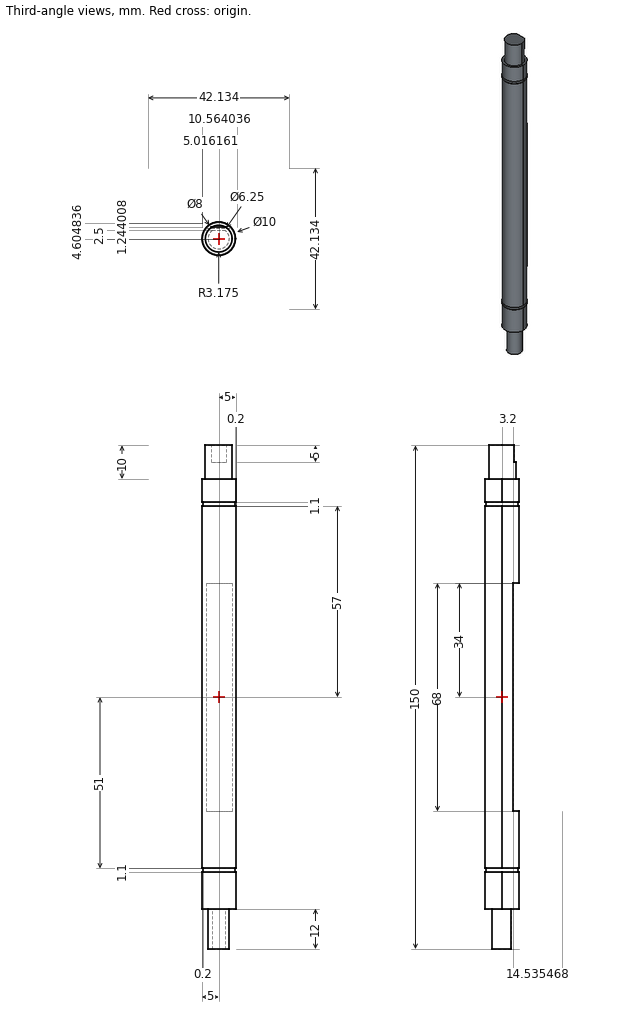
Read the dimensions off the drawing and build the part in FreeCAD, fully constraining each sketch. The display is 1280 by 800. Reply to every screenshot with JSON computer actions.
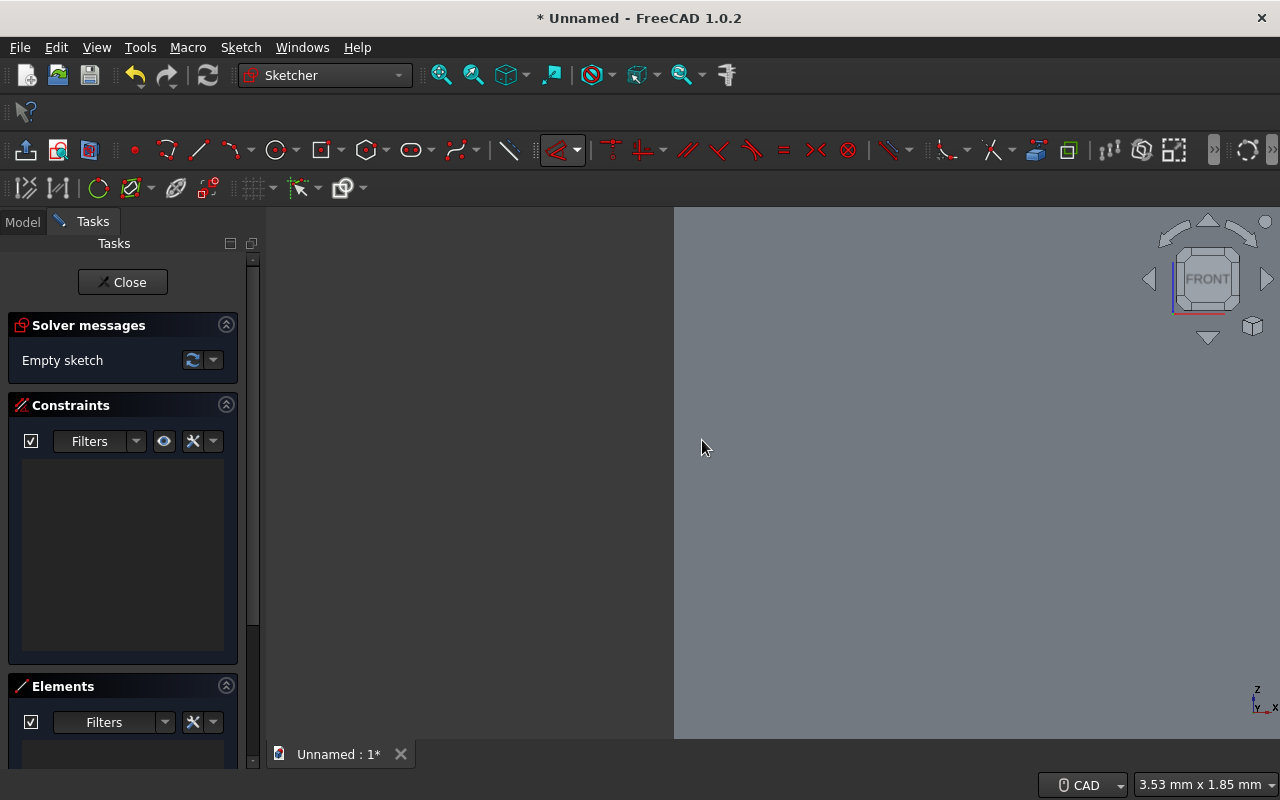
{"action": "left_click", "coordinate": [344, 150]}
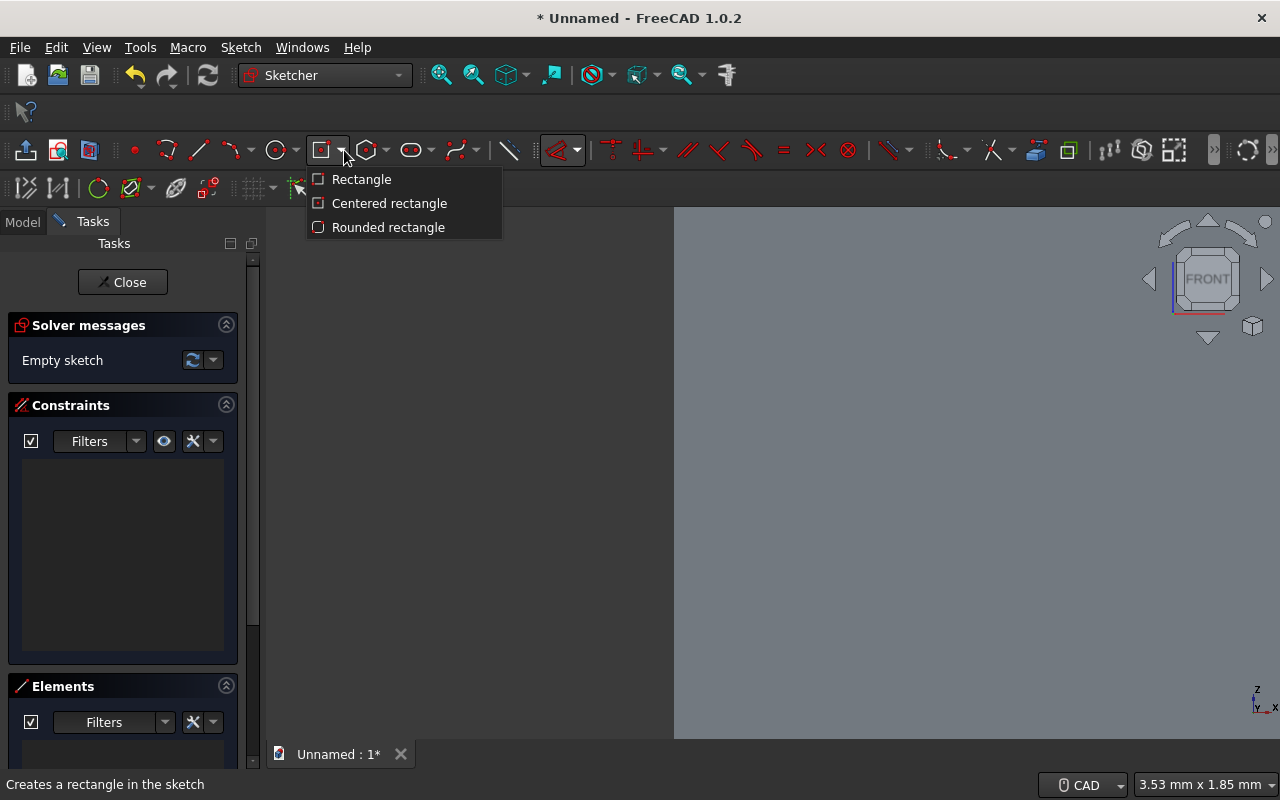
{"action": "left_click", "coordinate": [404, 179]}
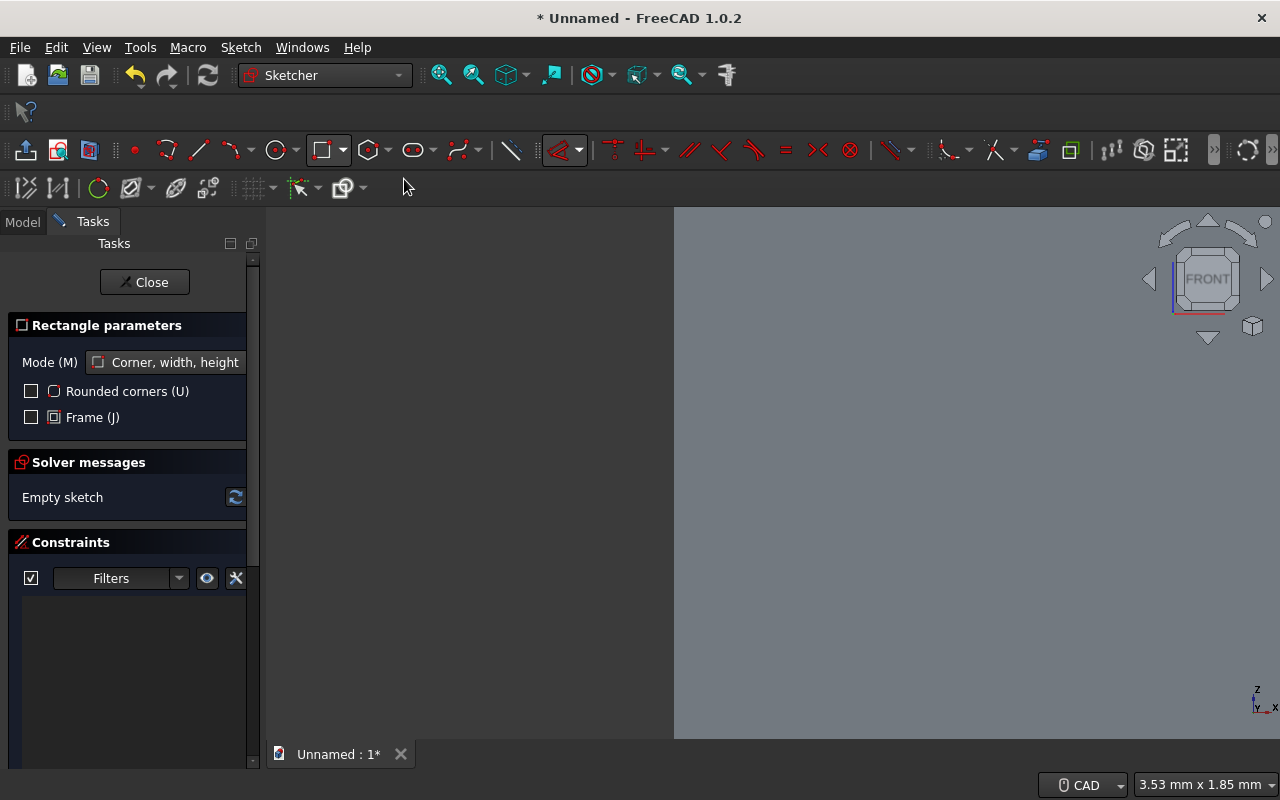
{"action": "left_click", "coordinate": [674, 314]}
{"action": "left_click", "coordinate": [731, 630]}
{"action": "key", "text": "Escape"}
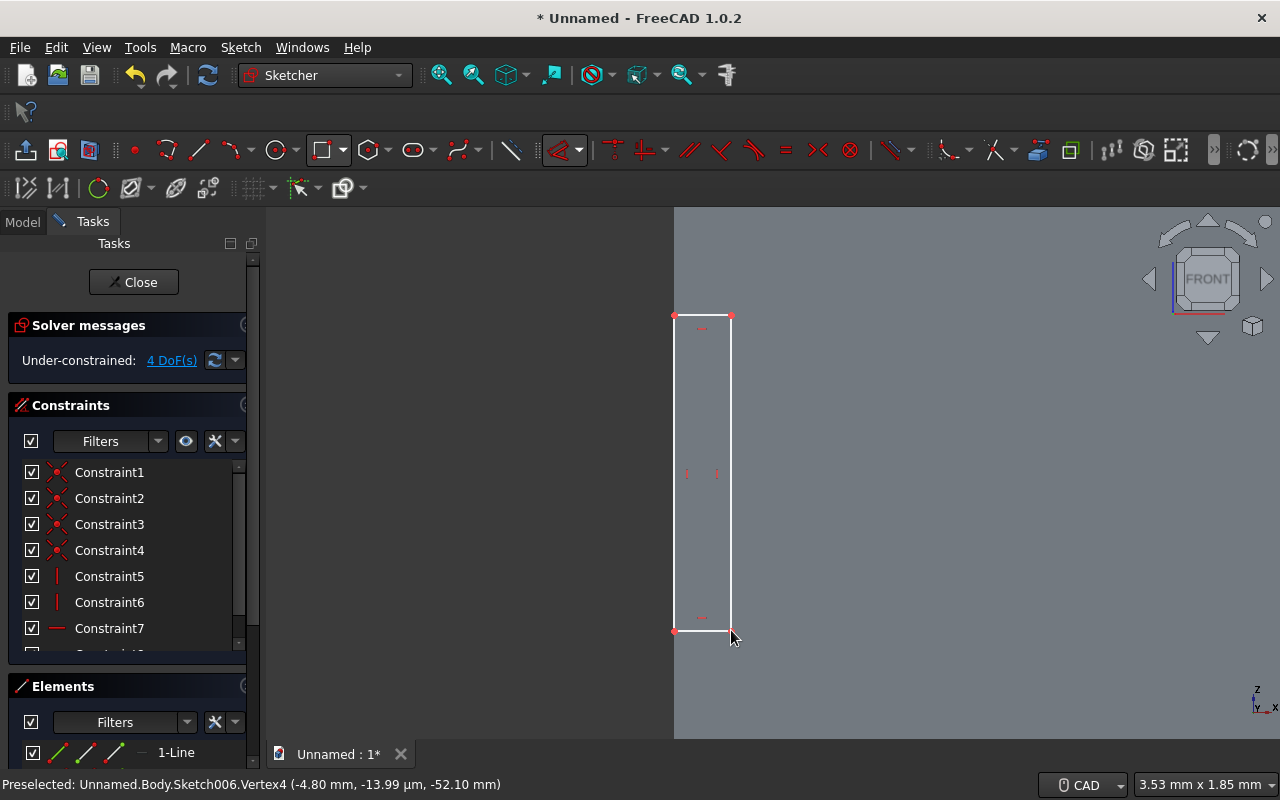
{"action": "left_click", "coordinate": [674, 315]}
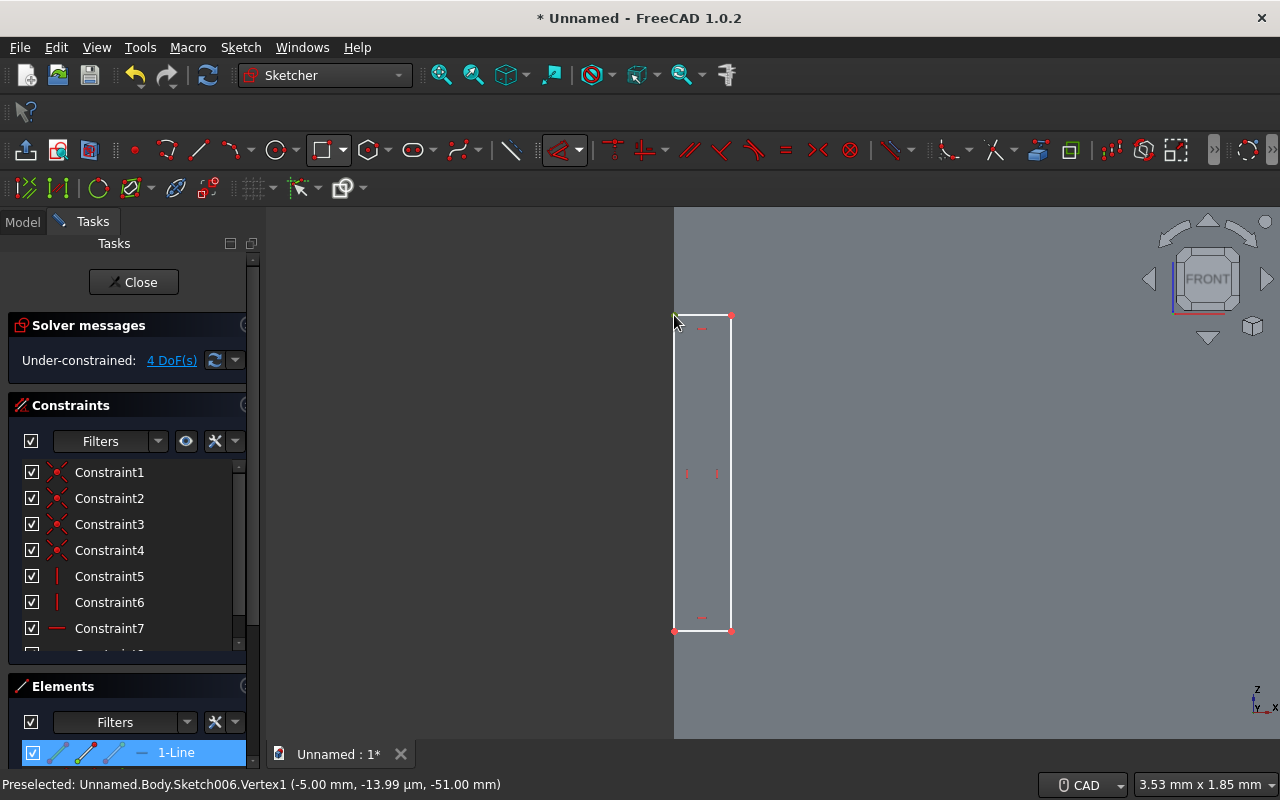
{"action": "left_click", "coordinate": [582, 150]}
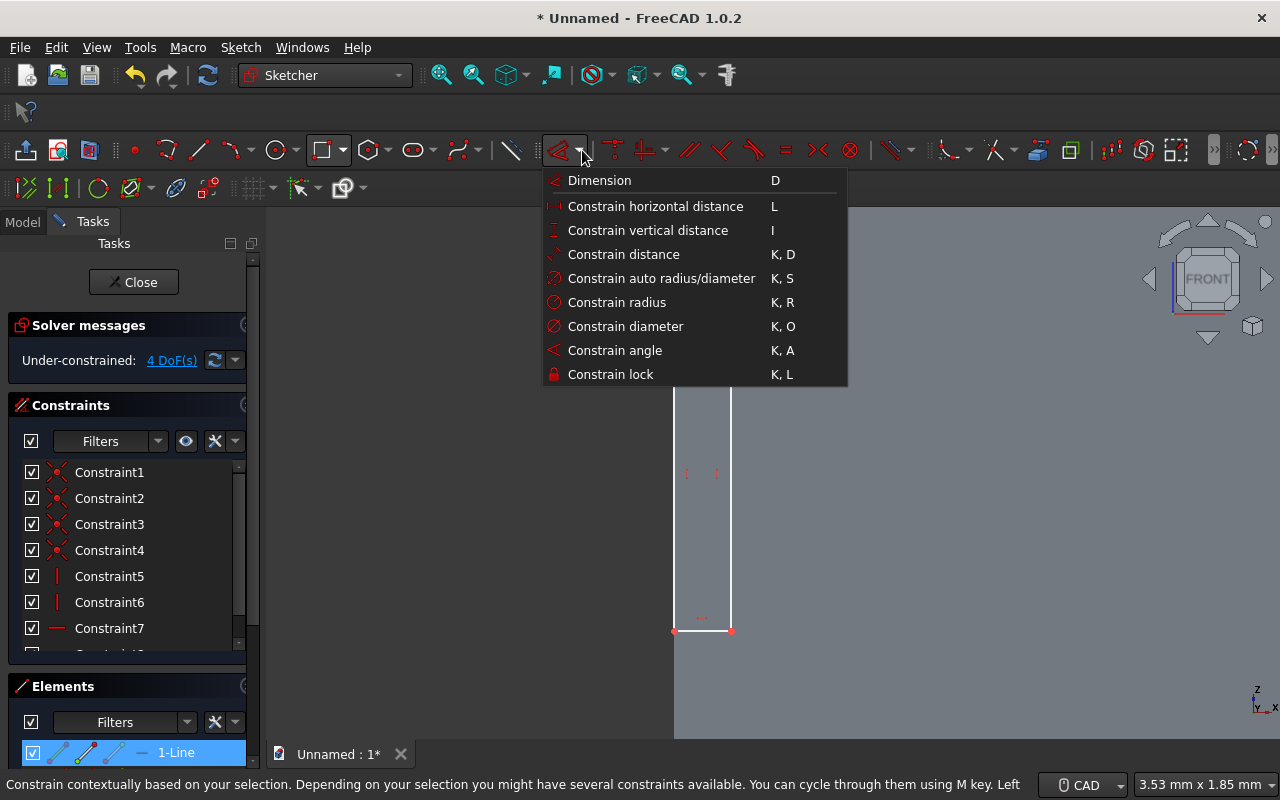
{"action": "left_click", "coordinate": [695, 206]}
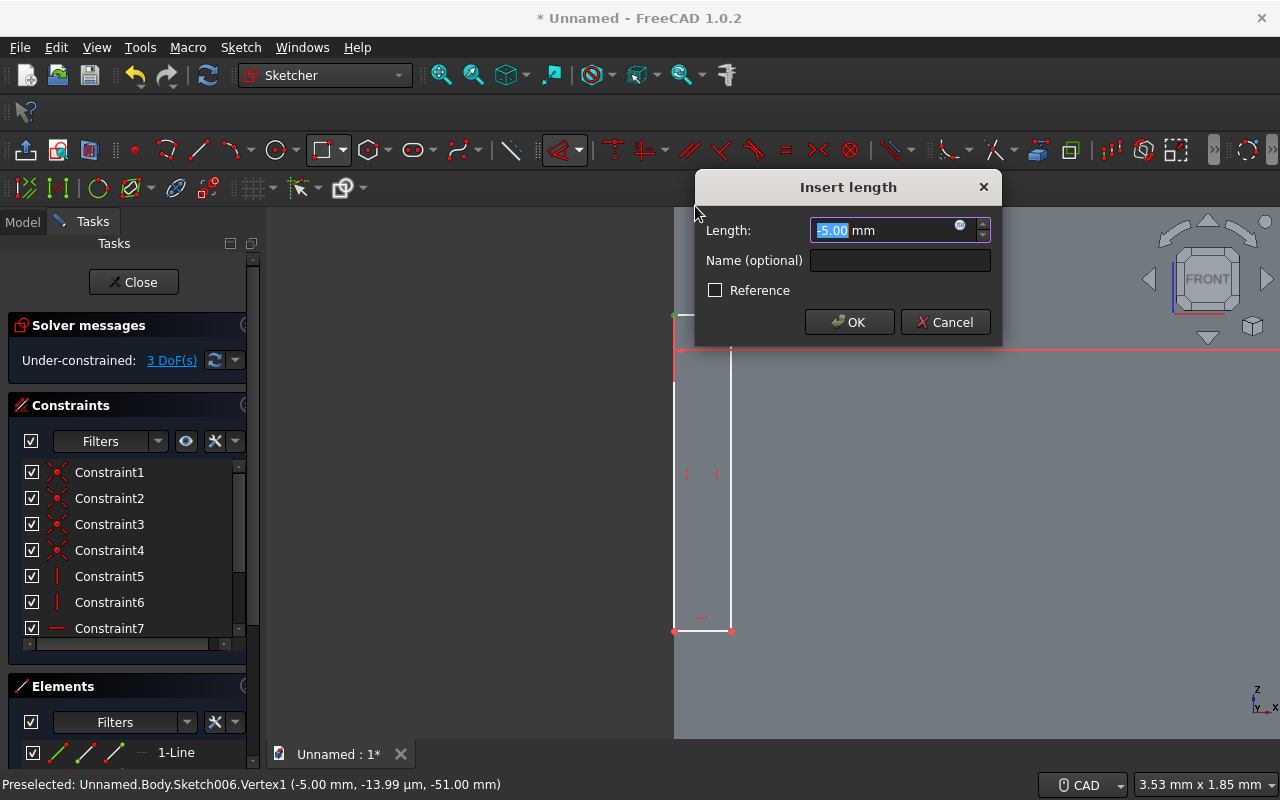
{"action": "type", "text": "-5"}
{"action": "key", "text": "Return"}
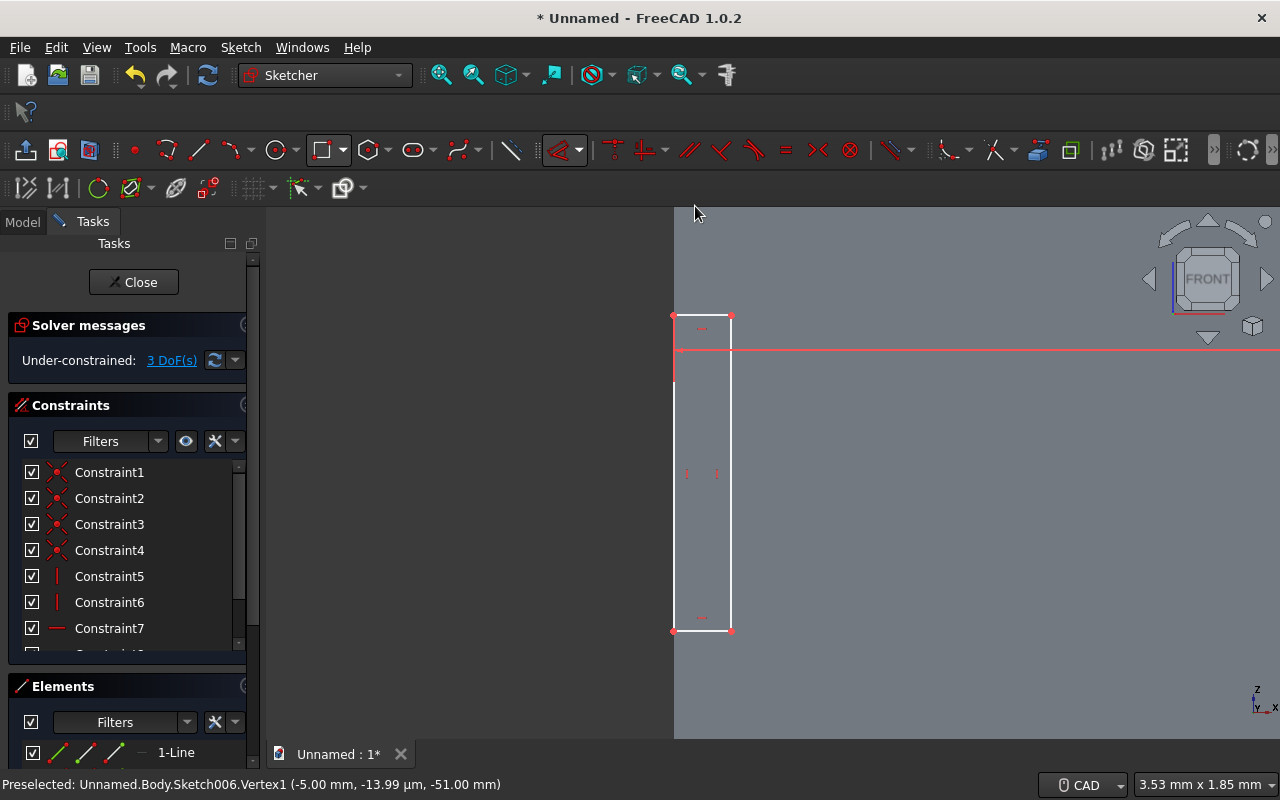
{"action": "left_click", "coordinate": [674, 410]}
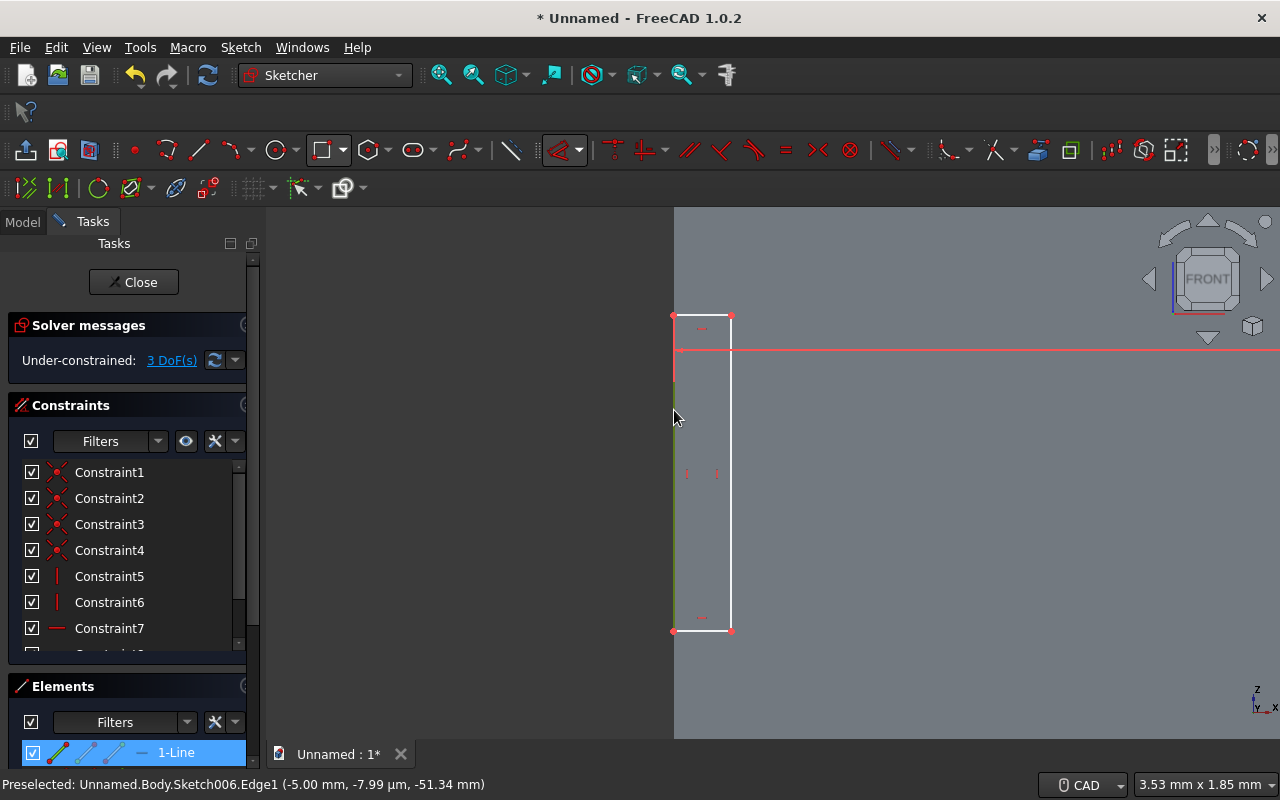
{"action": "key", "text": "i"}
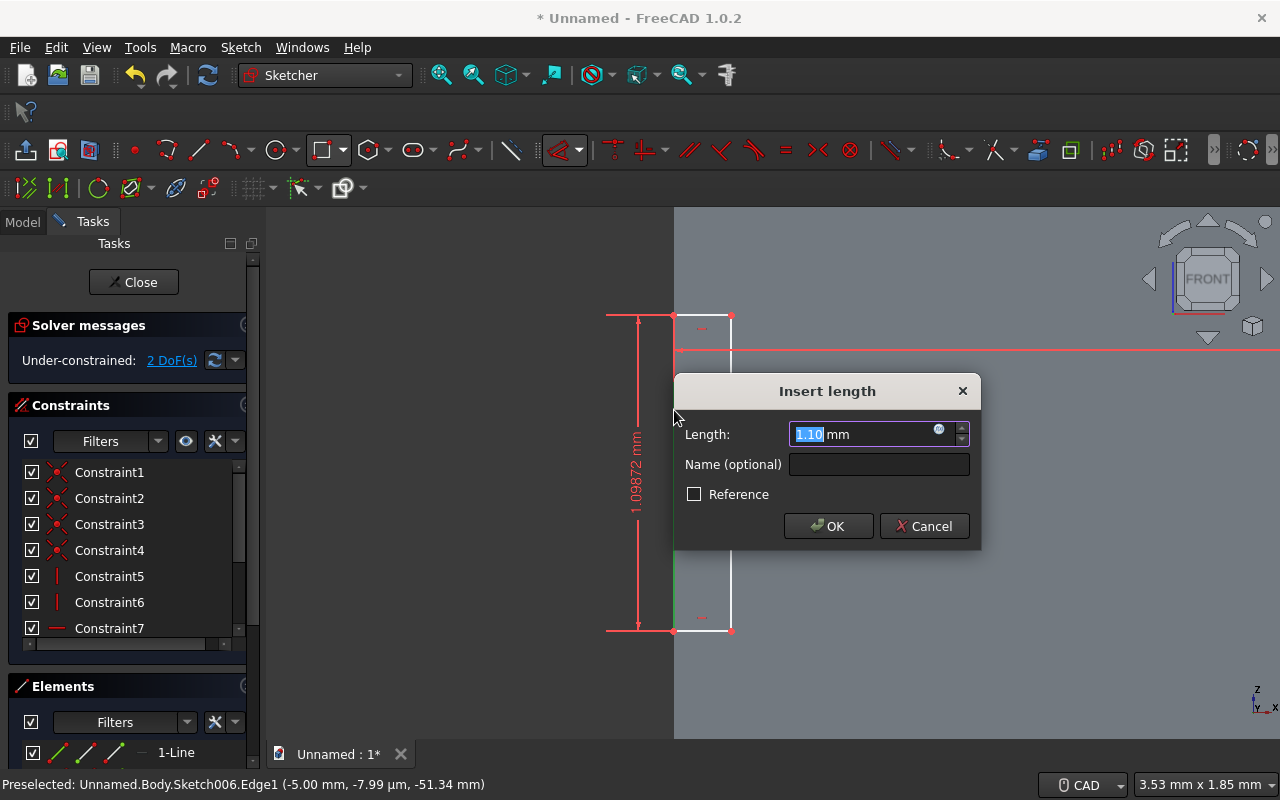
{"action": "type", "text": "1.1"}
{"action": "key", "text": "Return"}